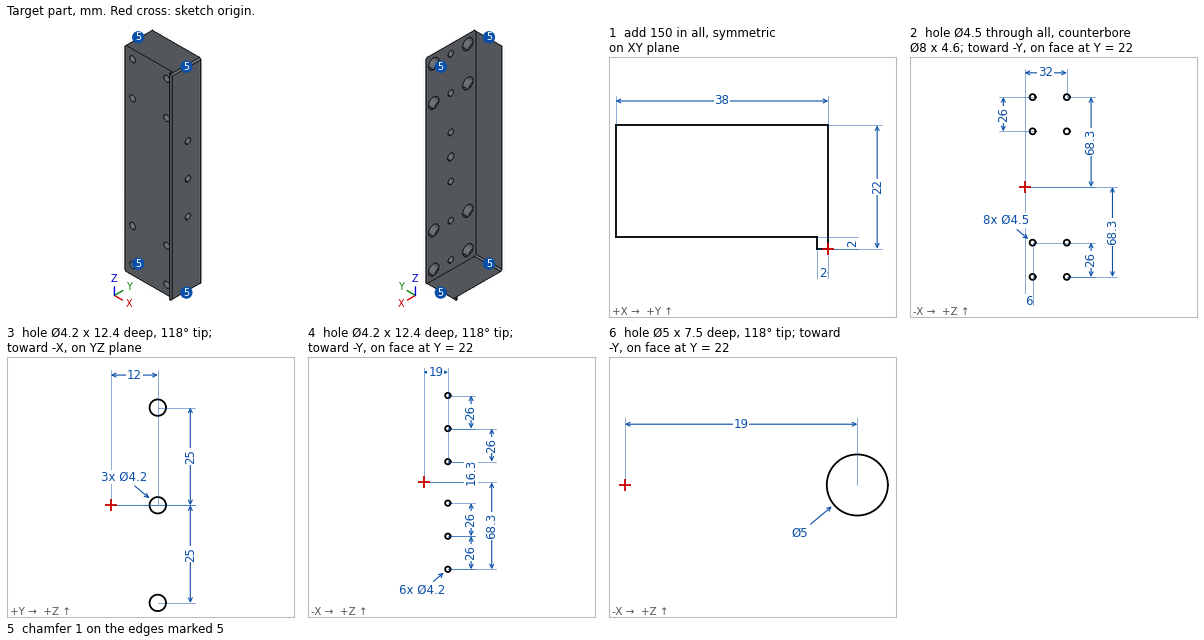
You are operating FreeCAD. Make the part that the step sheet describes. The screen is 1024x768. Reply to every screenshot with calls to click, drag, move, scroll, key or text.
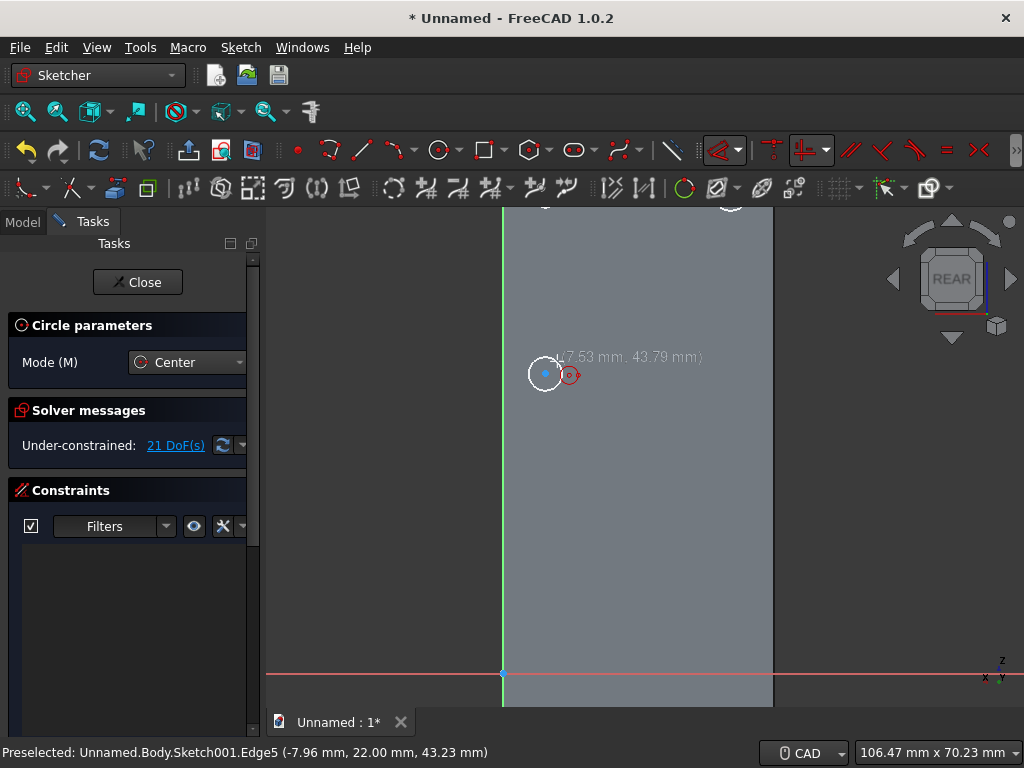
scroll(731, 373, up, 2)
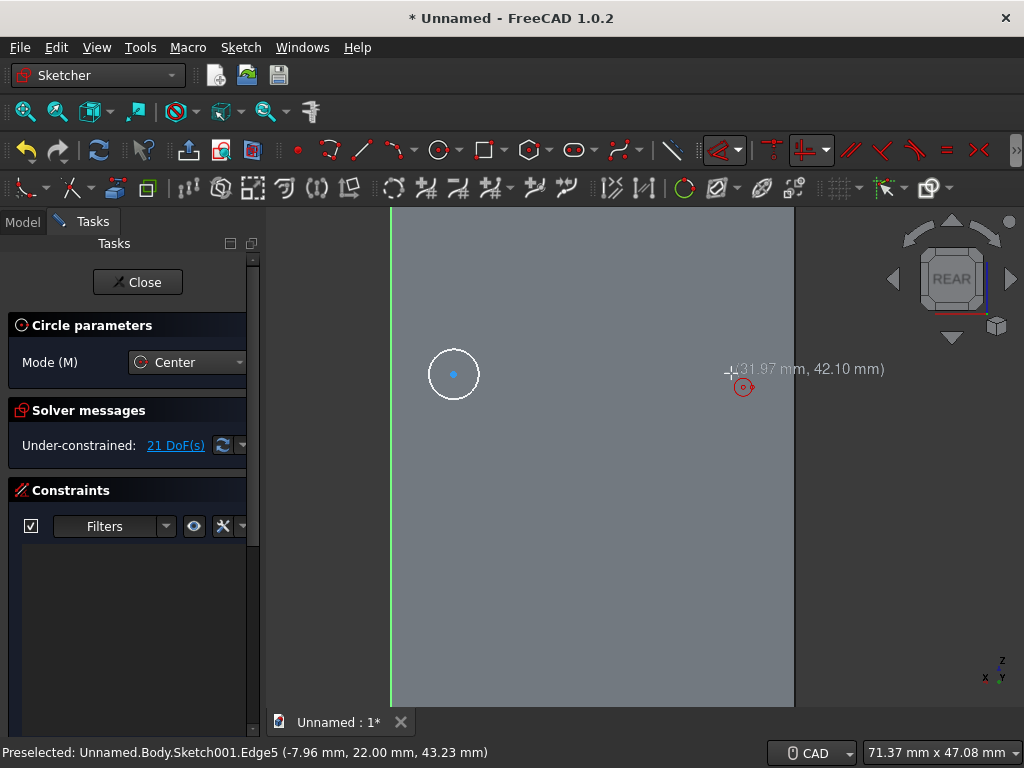
scroll(577, 365, down, 8)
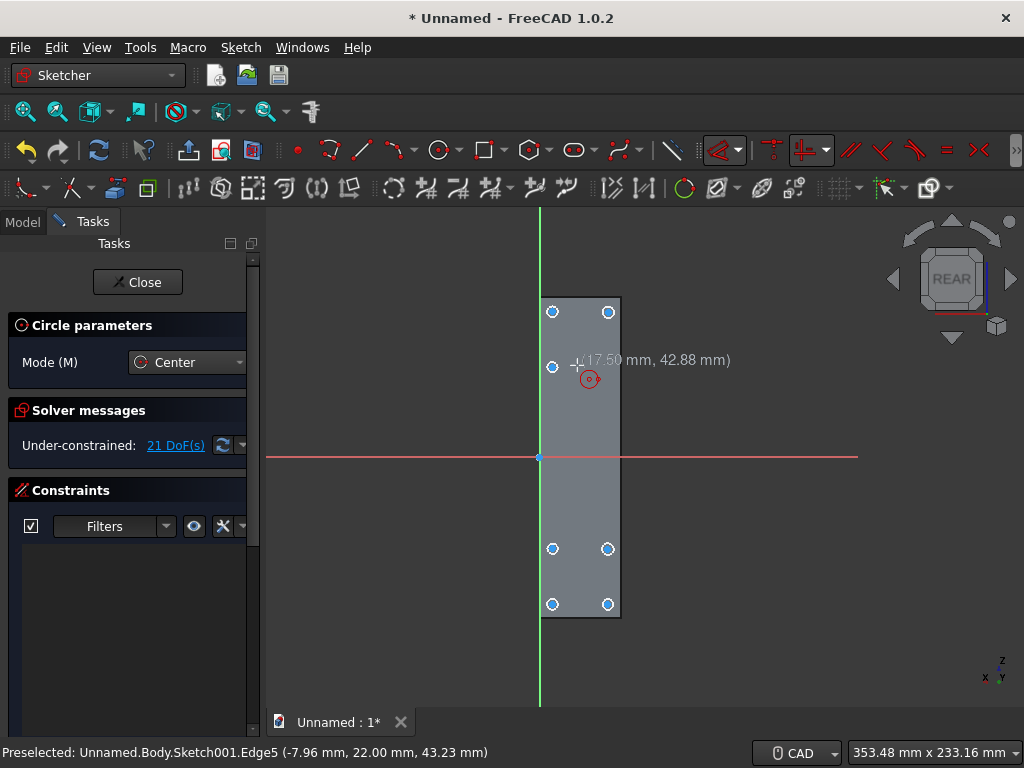
click(608, 367)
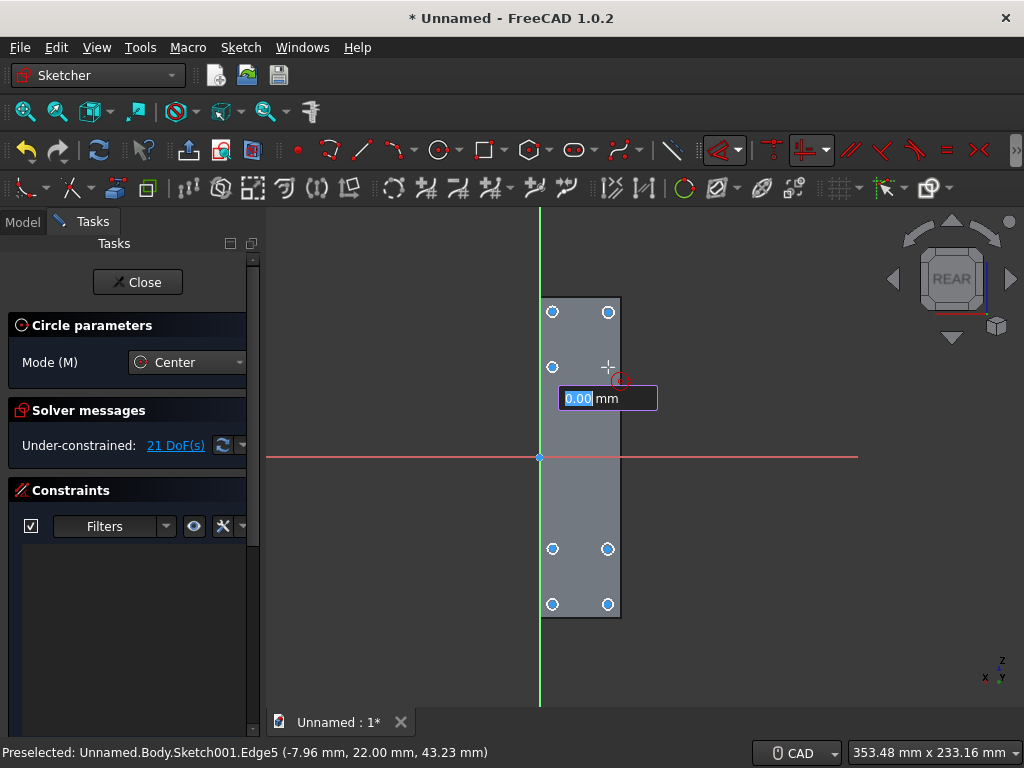
scroll(612, 363, up, 6)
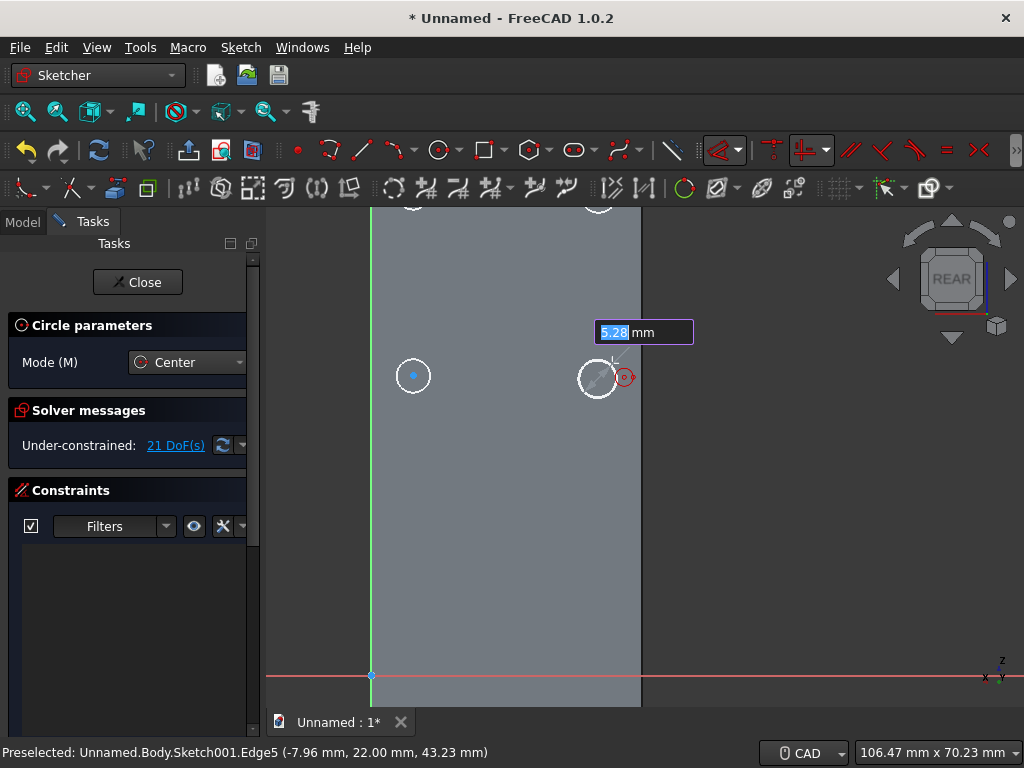
click(610, 363)
key(Escape)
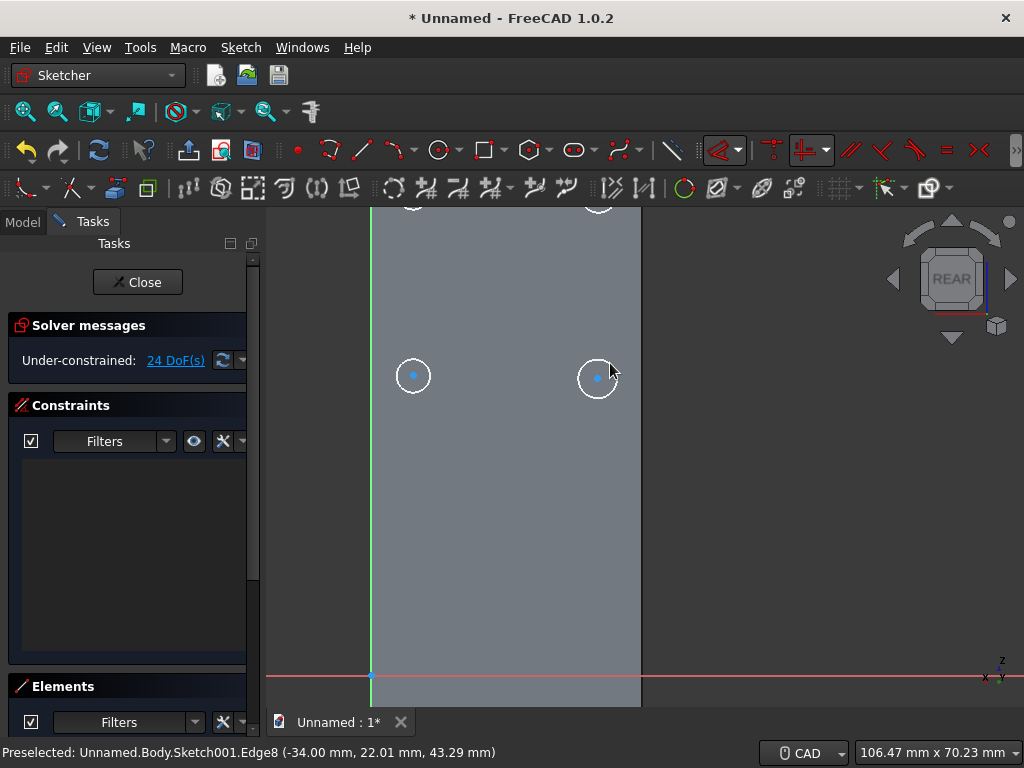
scroll(612, 363, down, 6)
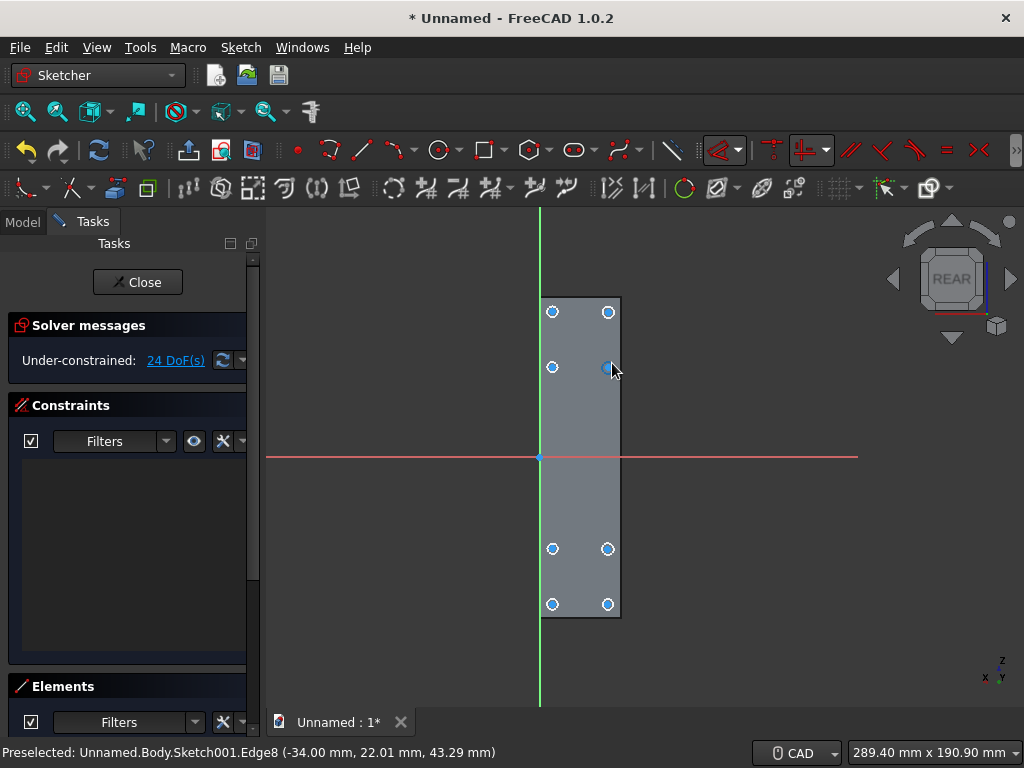
scroll(612, 308, up, 5)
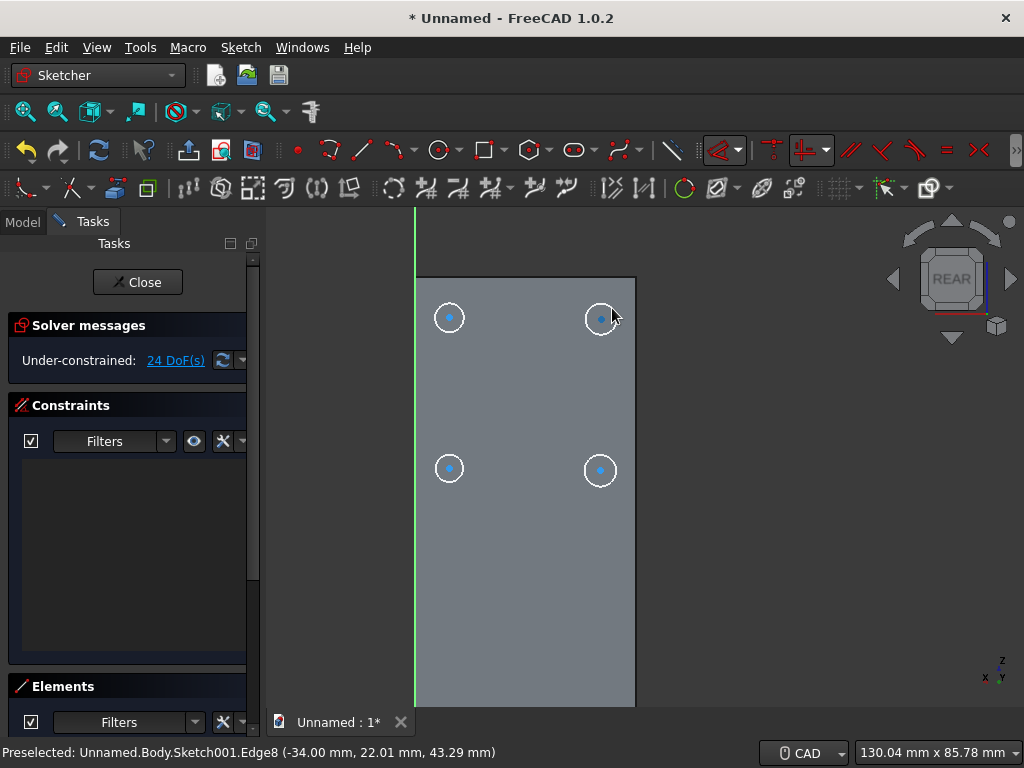
click(612, 308)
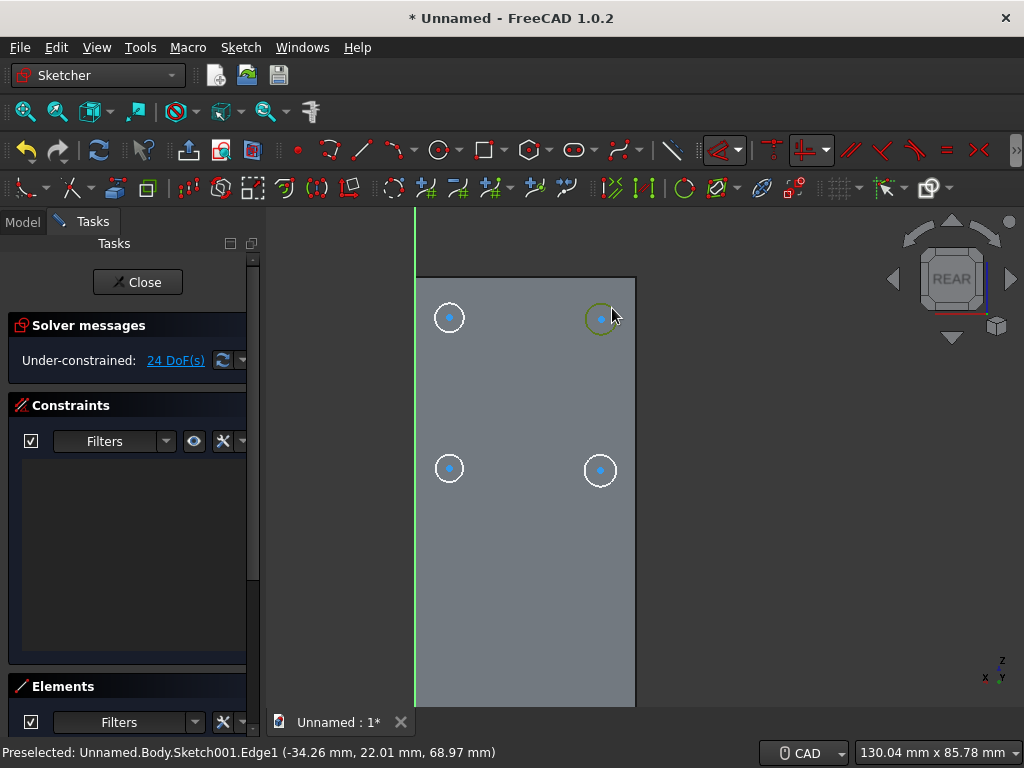
scroll(612, 308, down, 5)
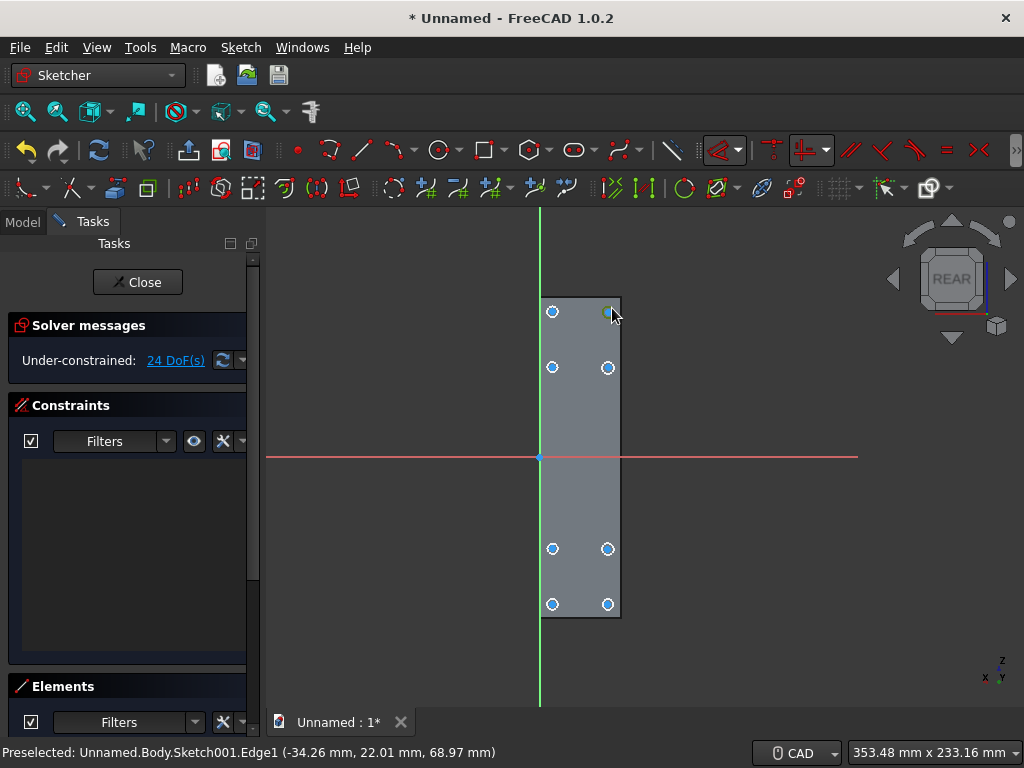
scroll(612, 601, up, 5)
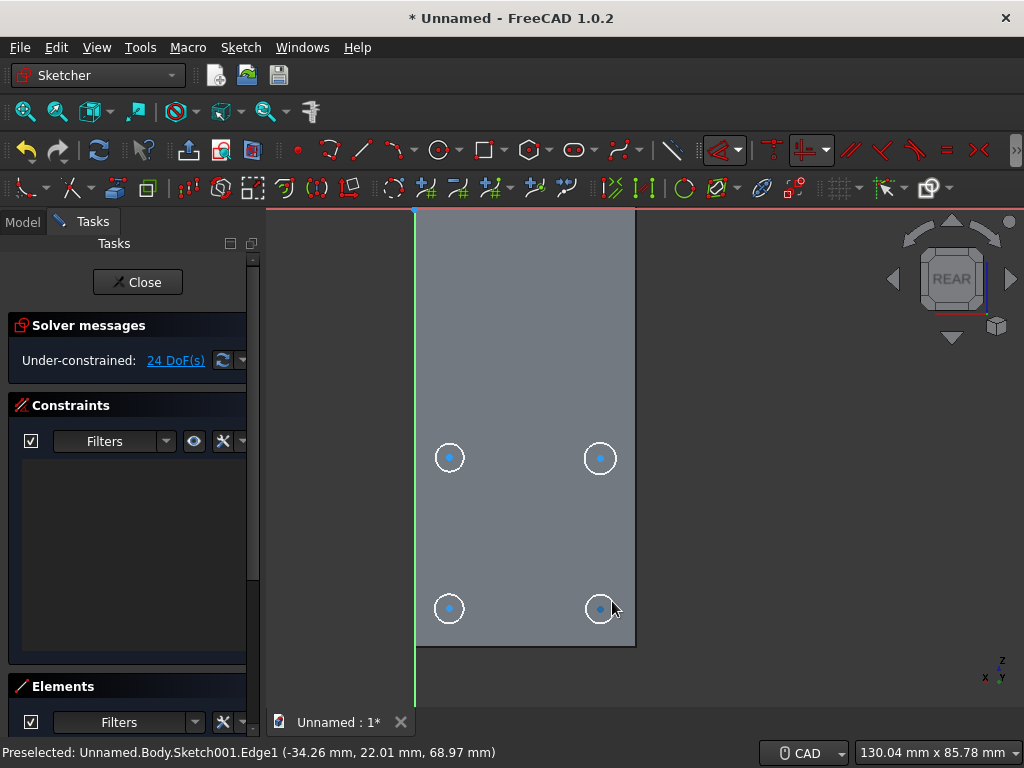
click(610, 599)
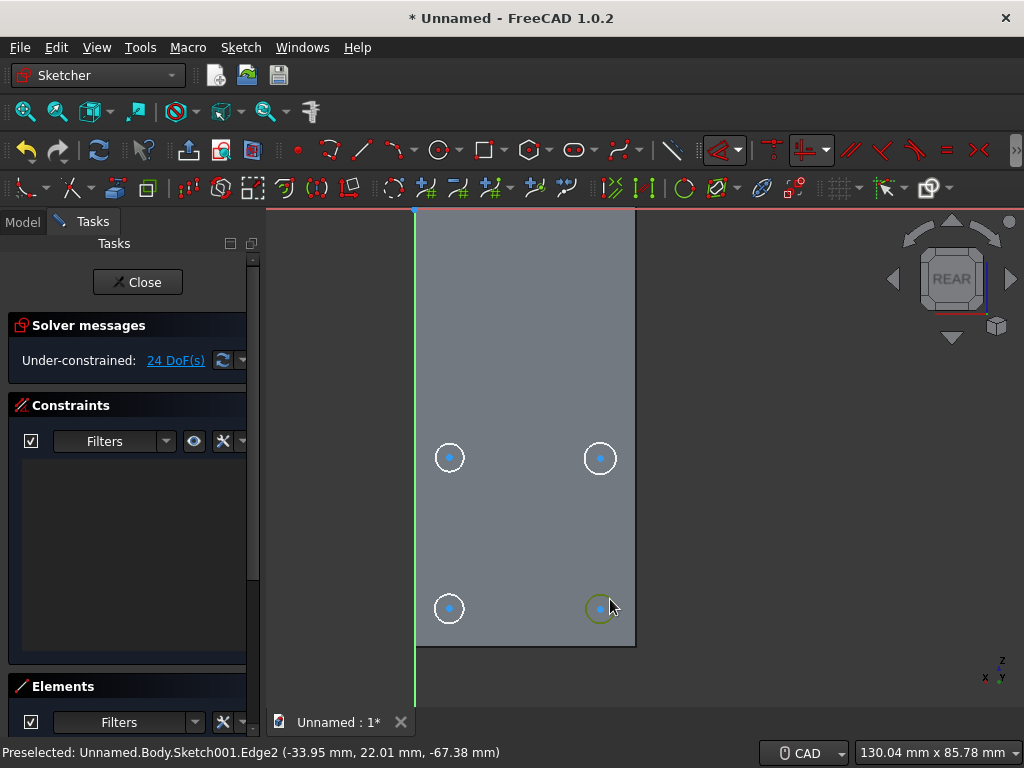
click(460, 448)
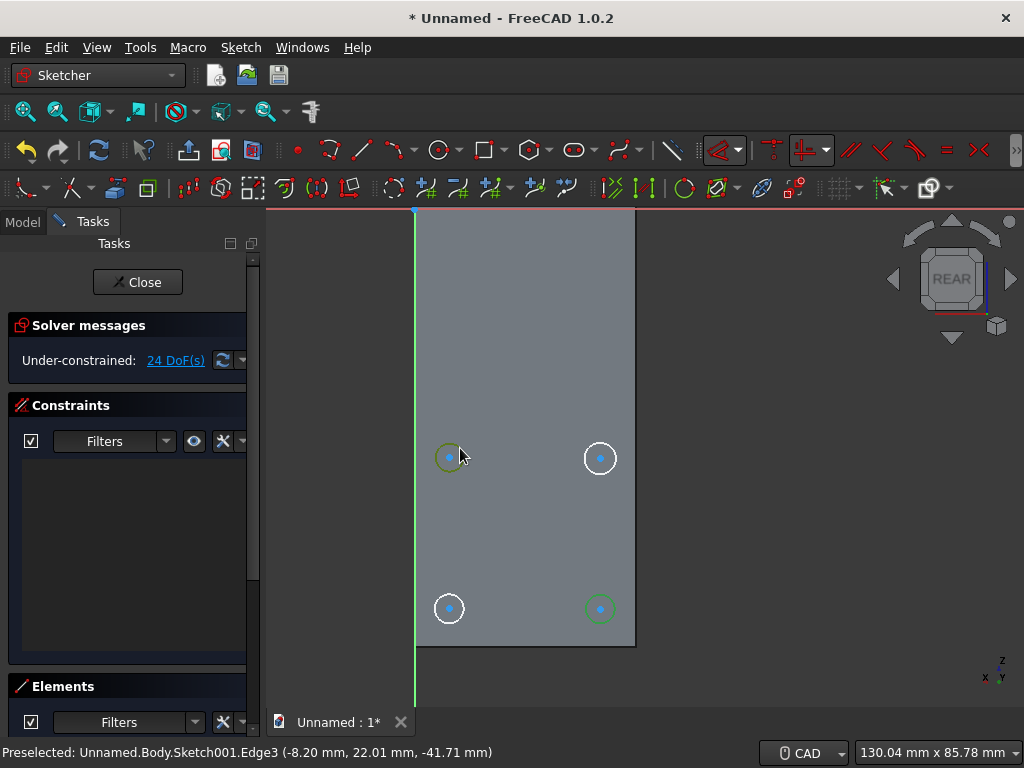
click(611, 447)